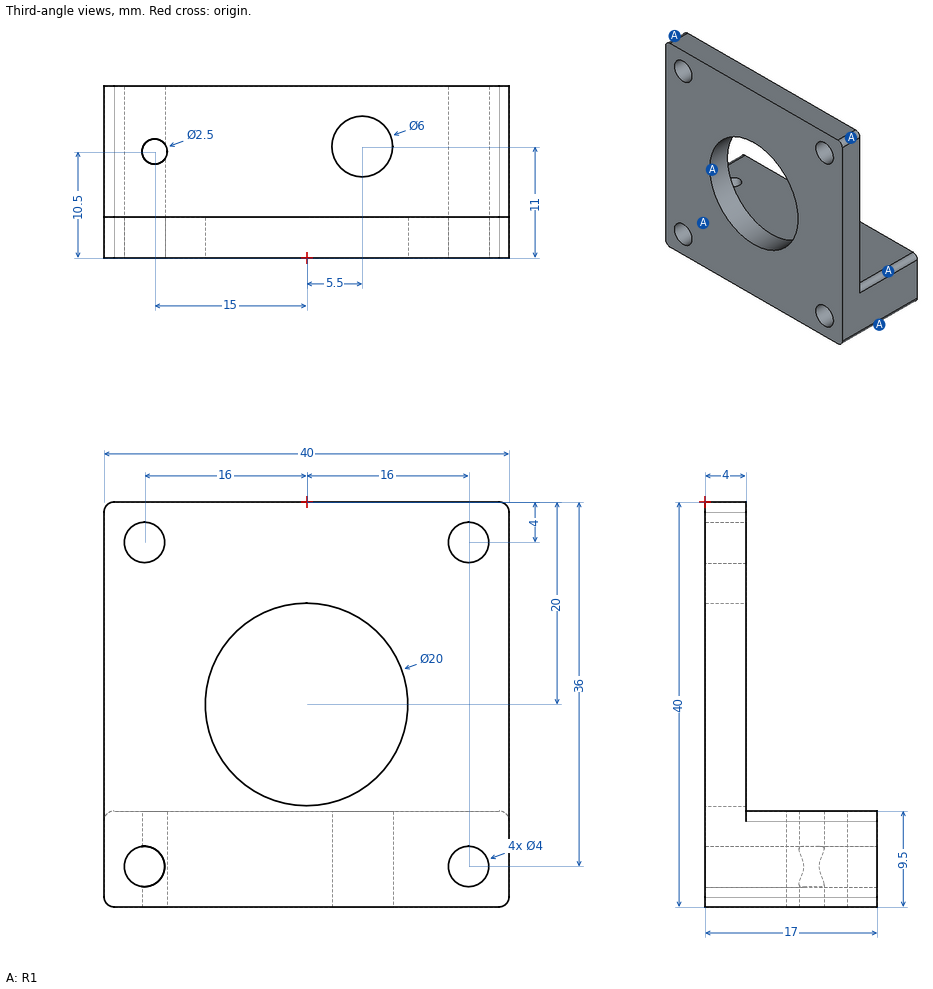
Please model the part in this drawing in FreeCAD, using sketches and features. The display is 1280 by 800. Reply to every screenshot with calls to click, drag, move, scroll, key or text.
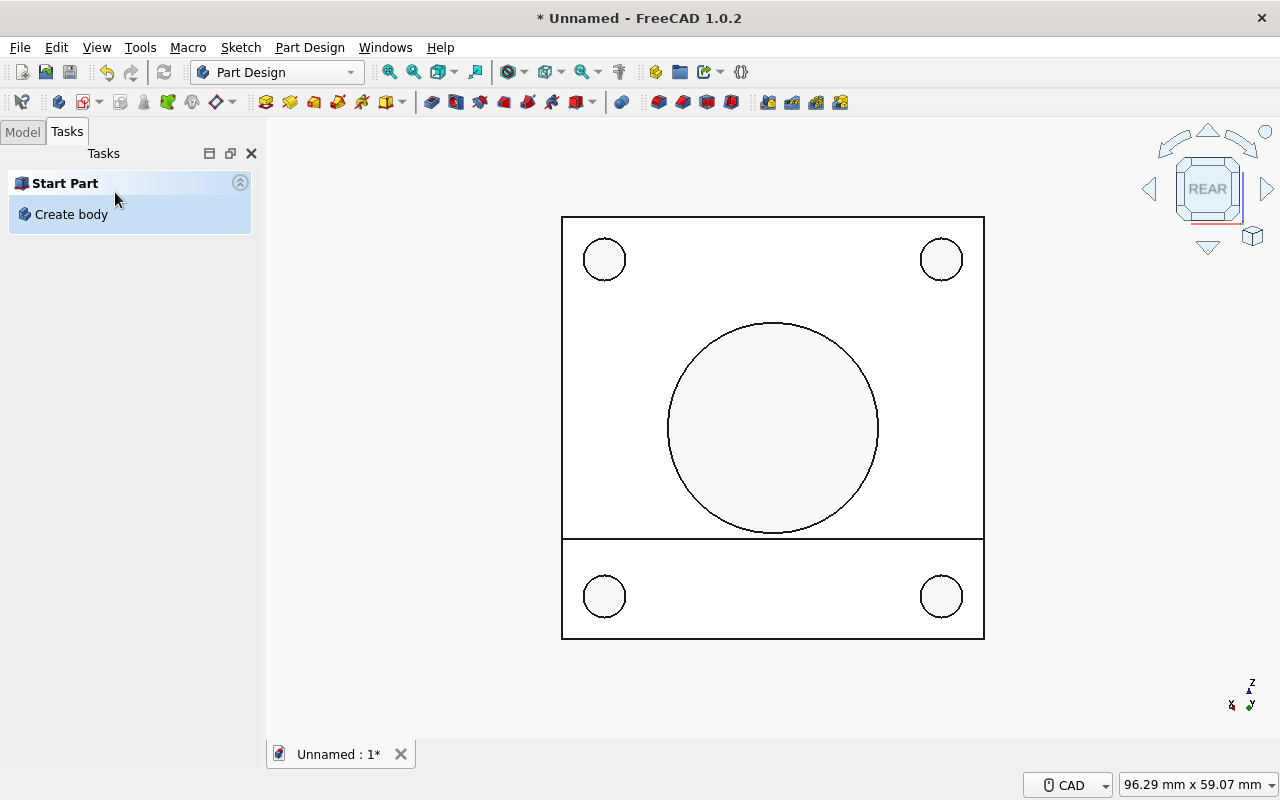
key(0)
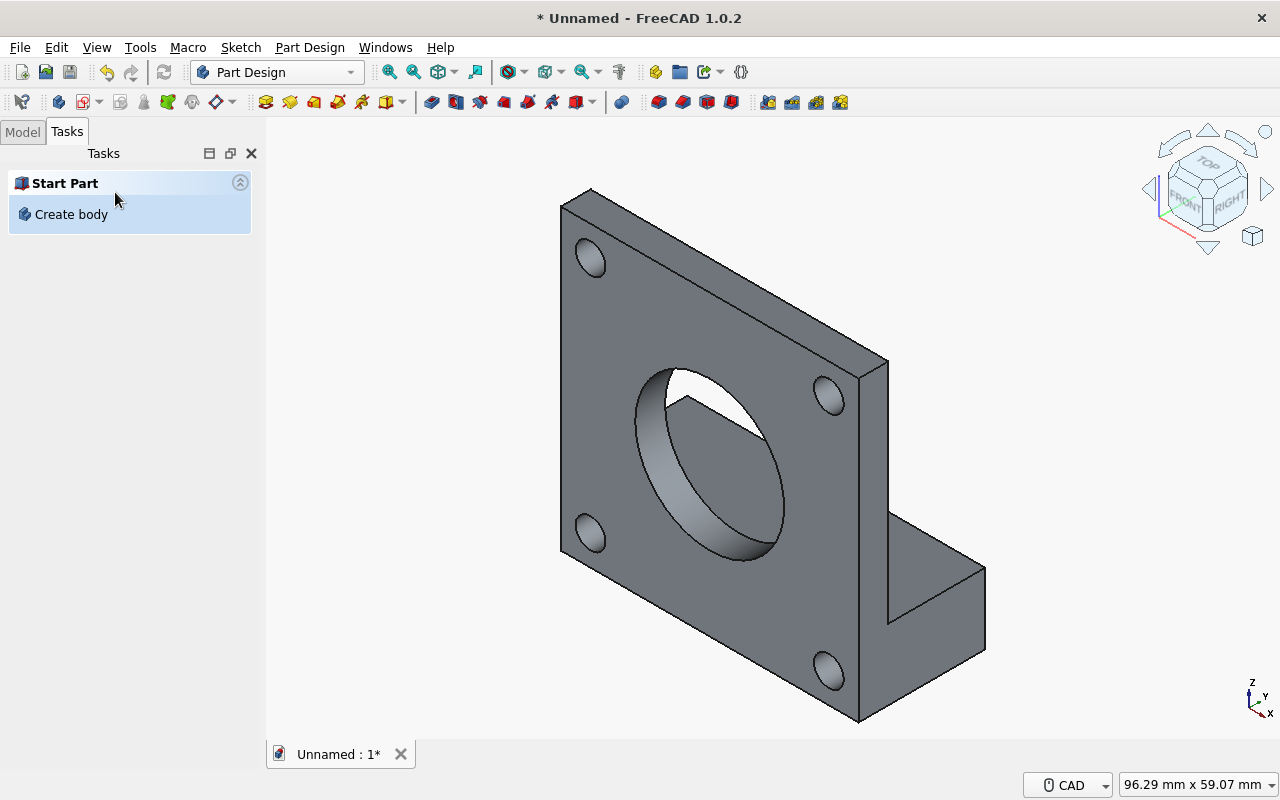
click(937, 595)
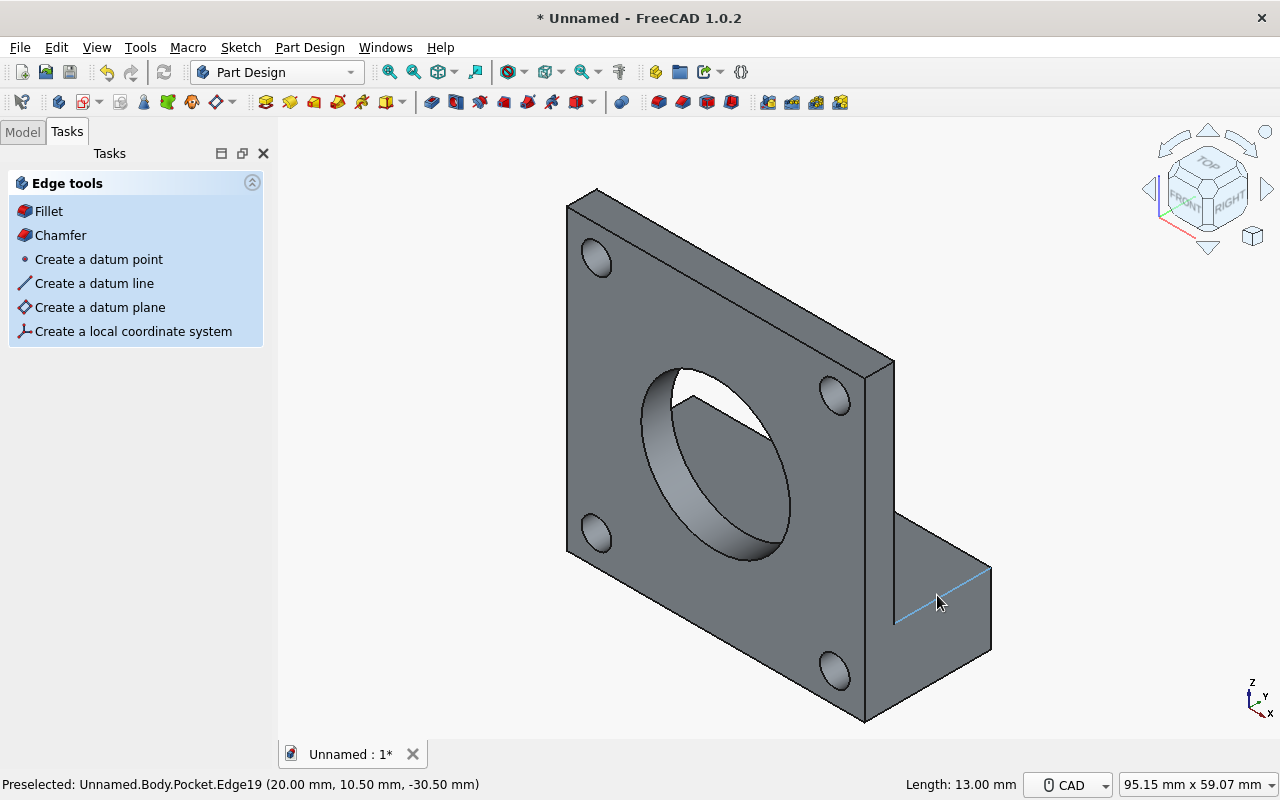
click(880, 369, ctrl)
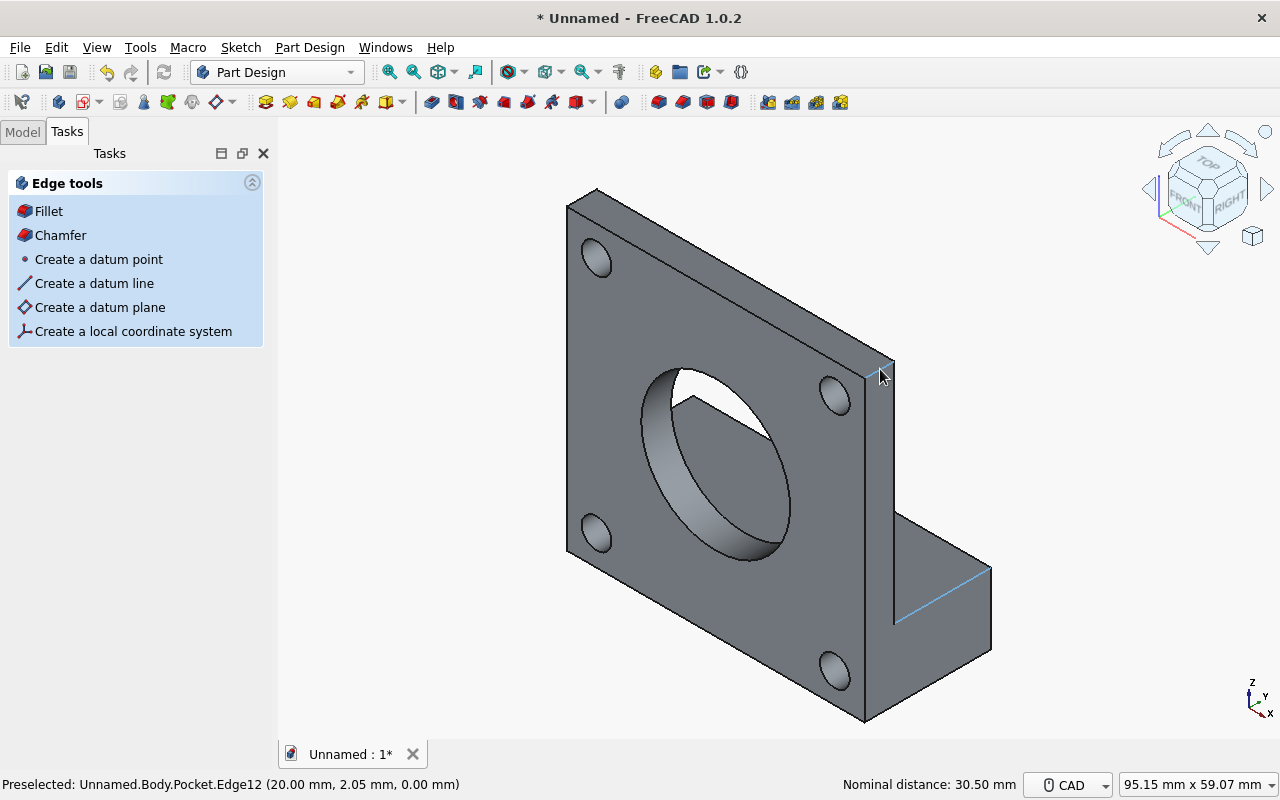
key(2)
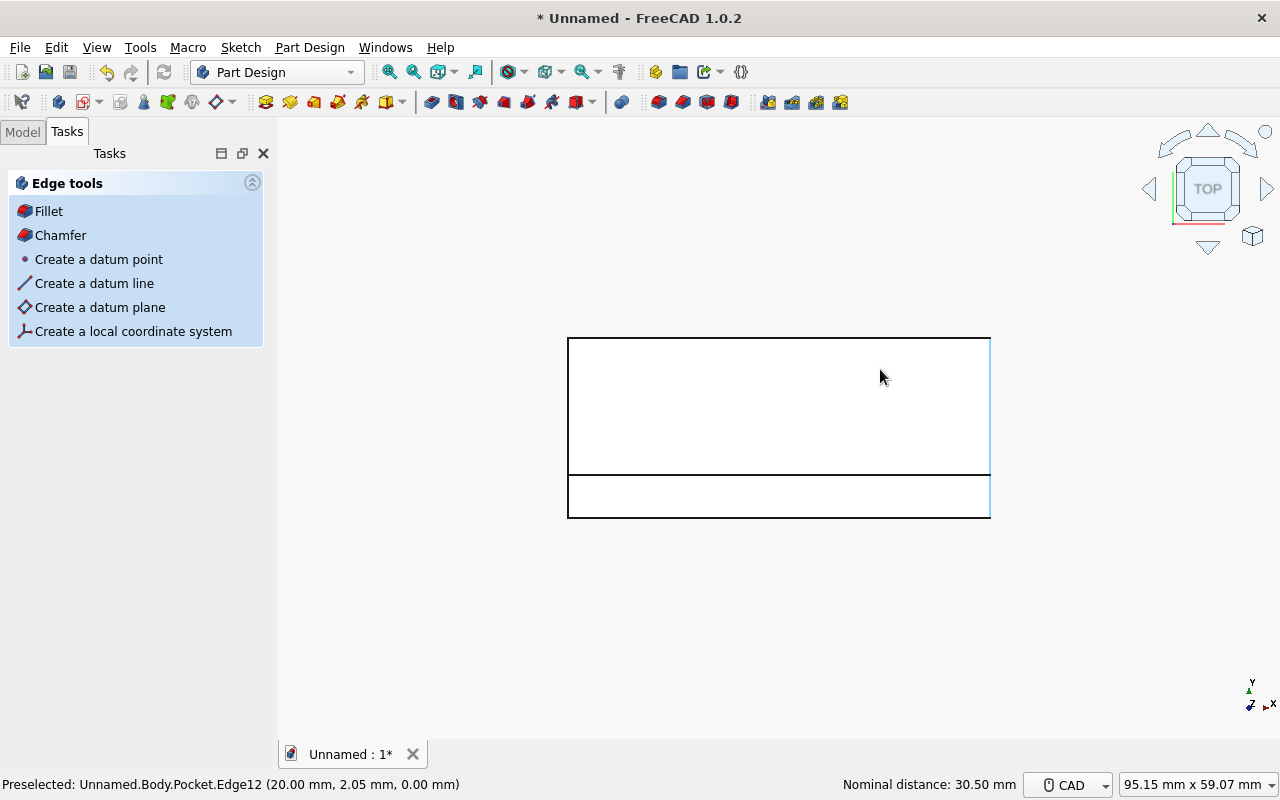
key(v)
key(f)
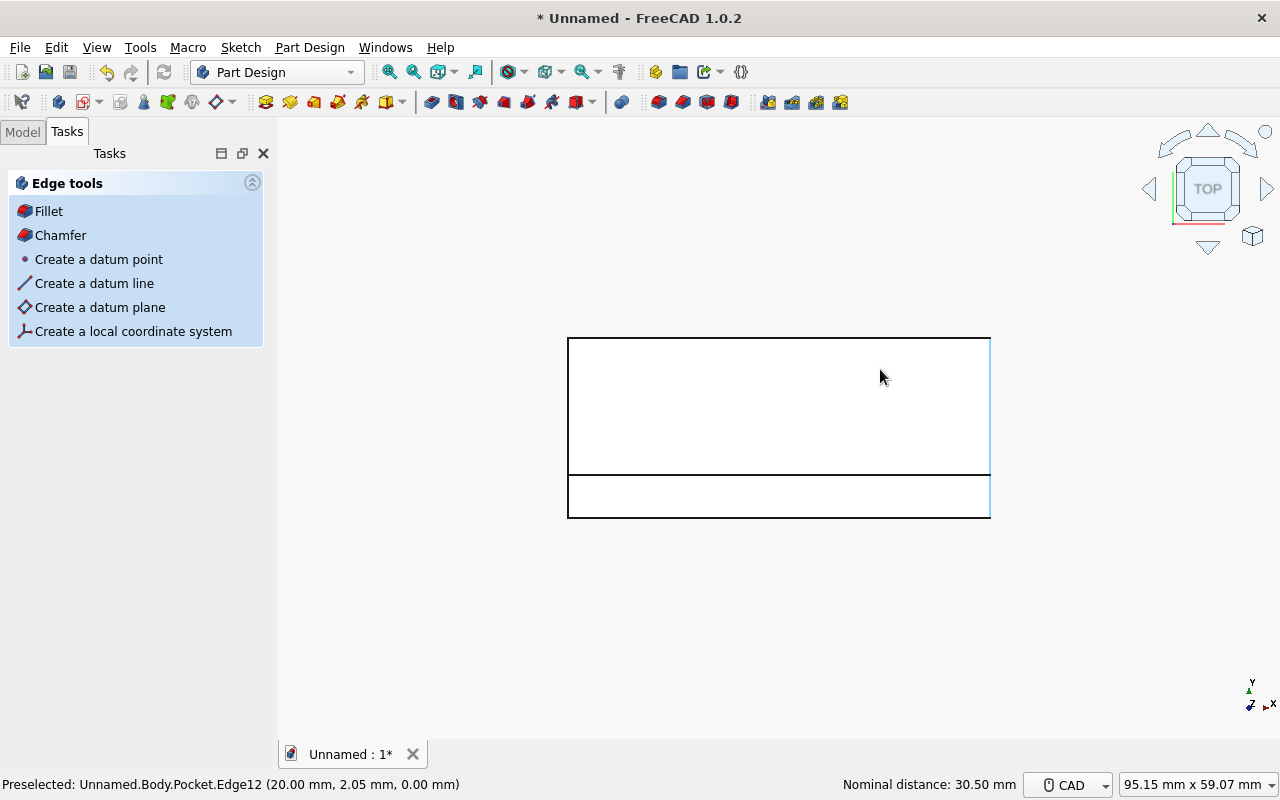
click(568, 406, ctrl)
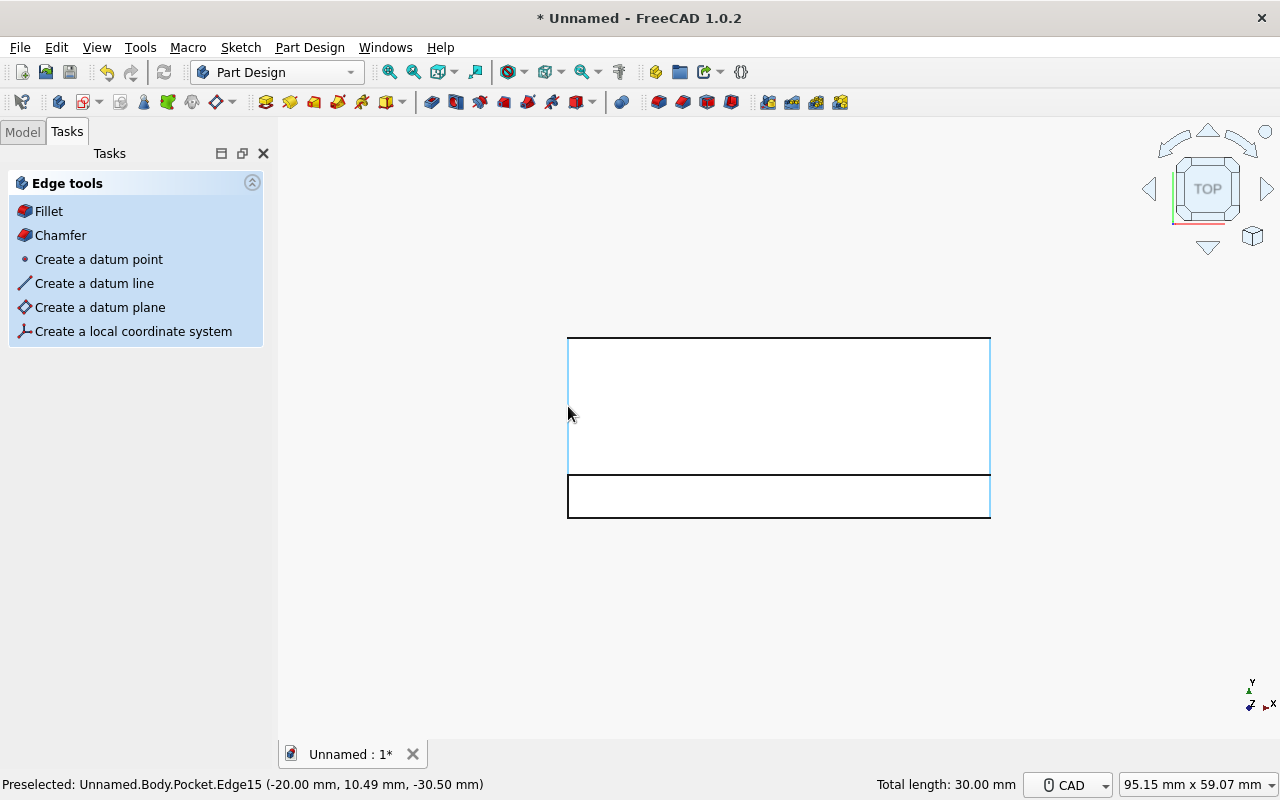
key(1)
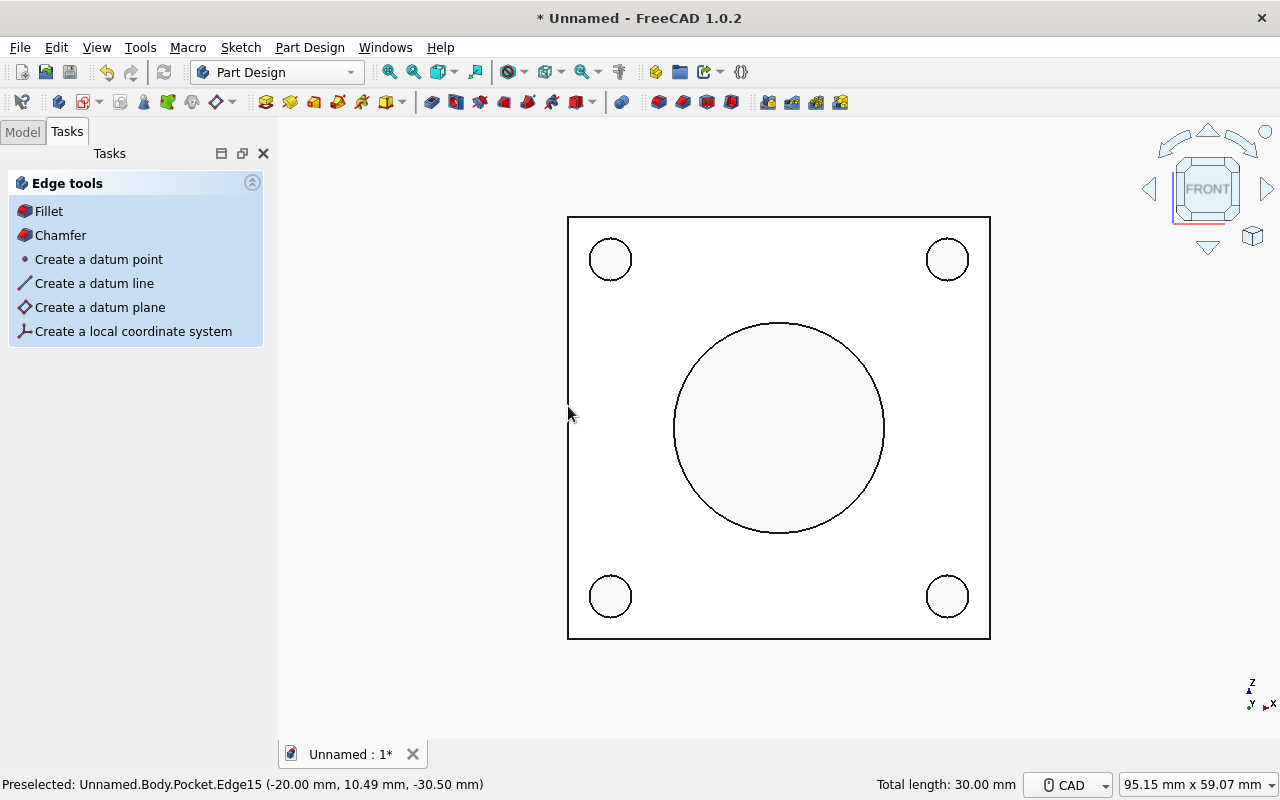
key(3)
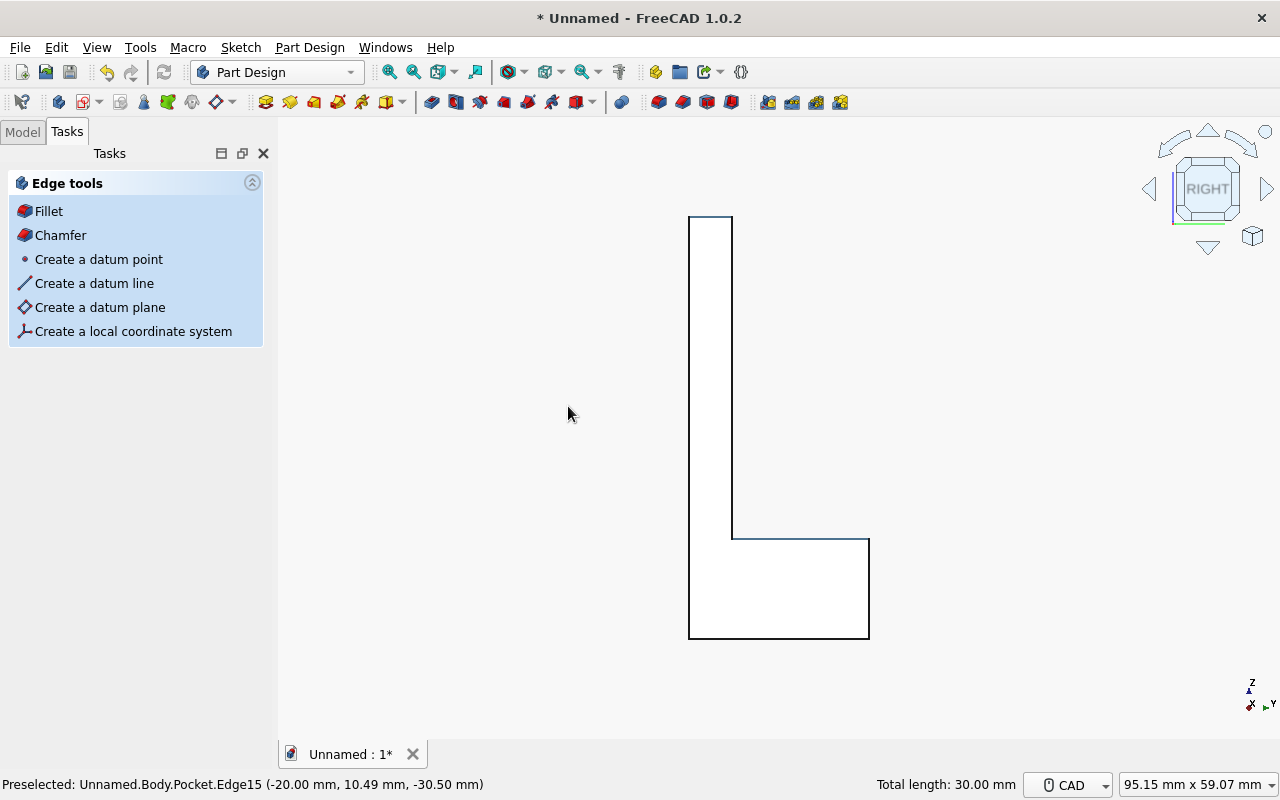
click(779, 638, ctrl)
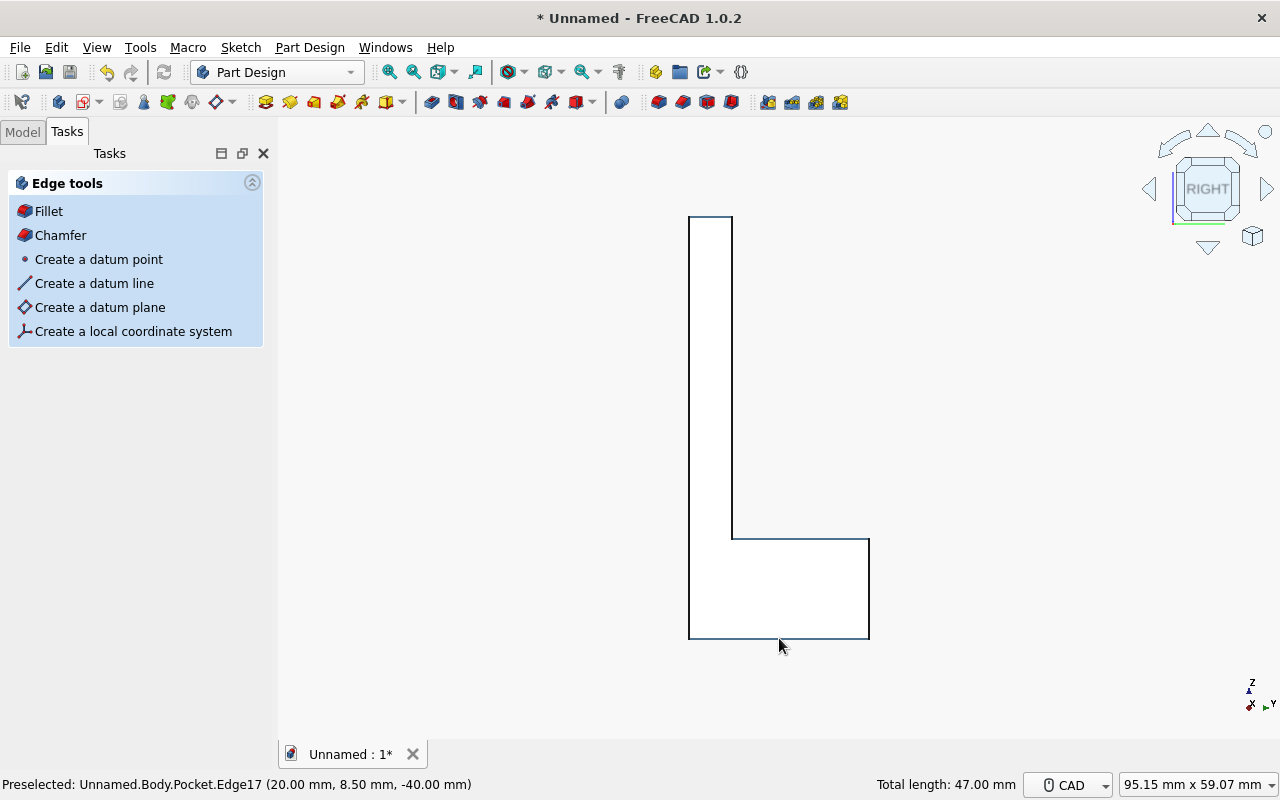
key(5)